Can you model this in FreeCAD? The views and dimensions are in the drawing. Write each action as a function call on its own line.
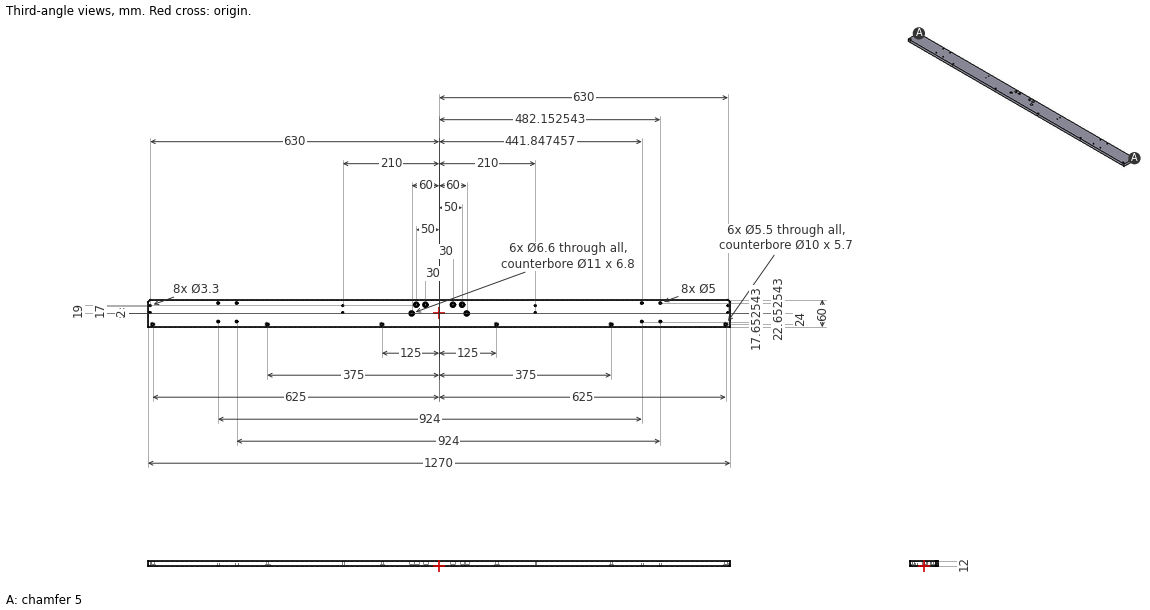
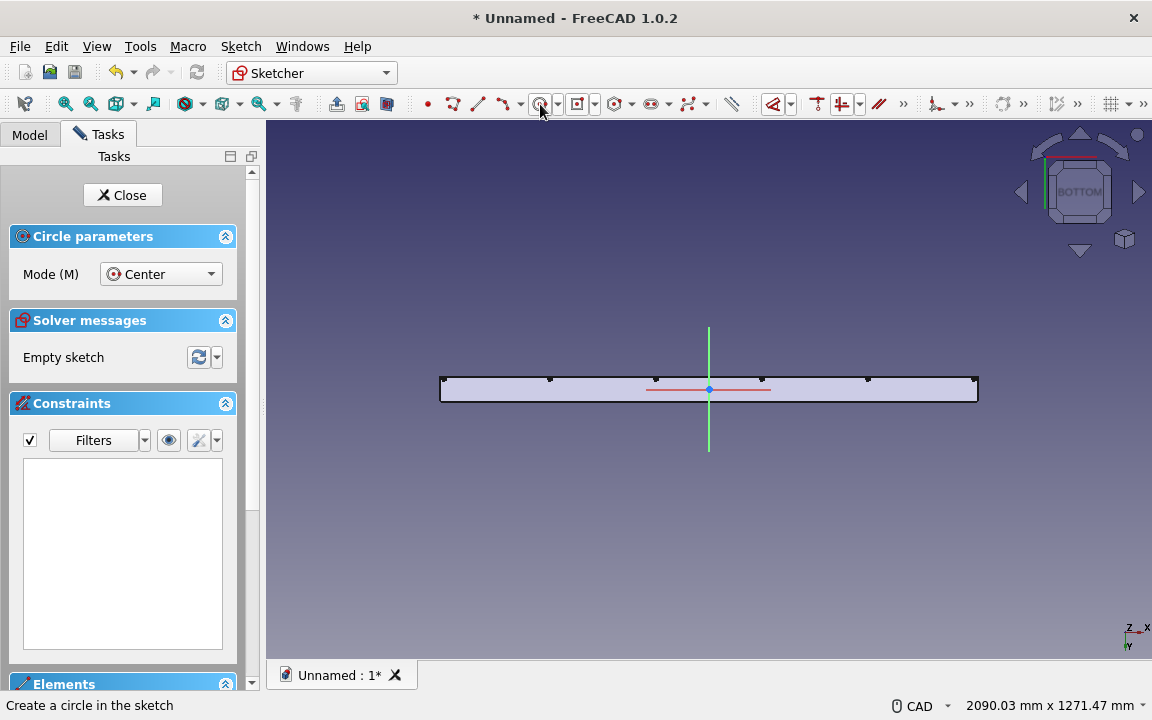
scroll(913, 399, up, 16)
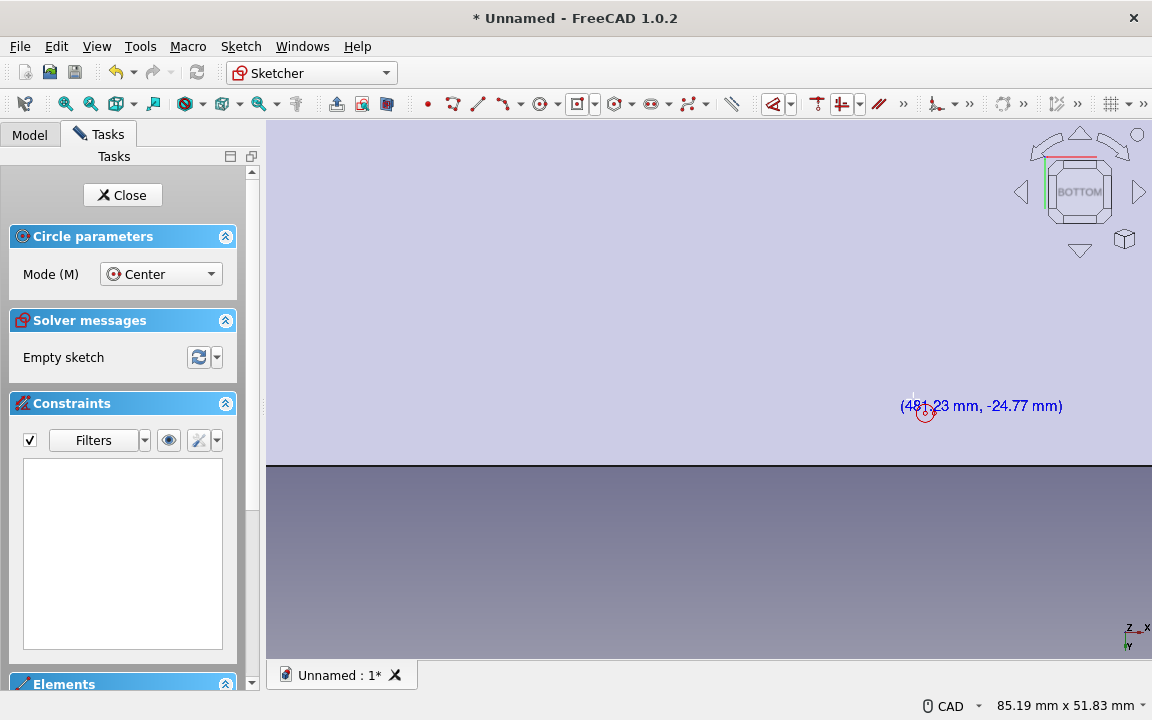
scroll(889, 400, down, 15)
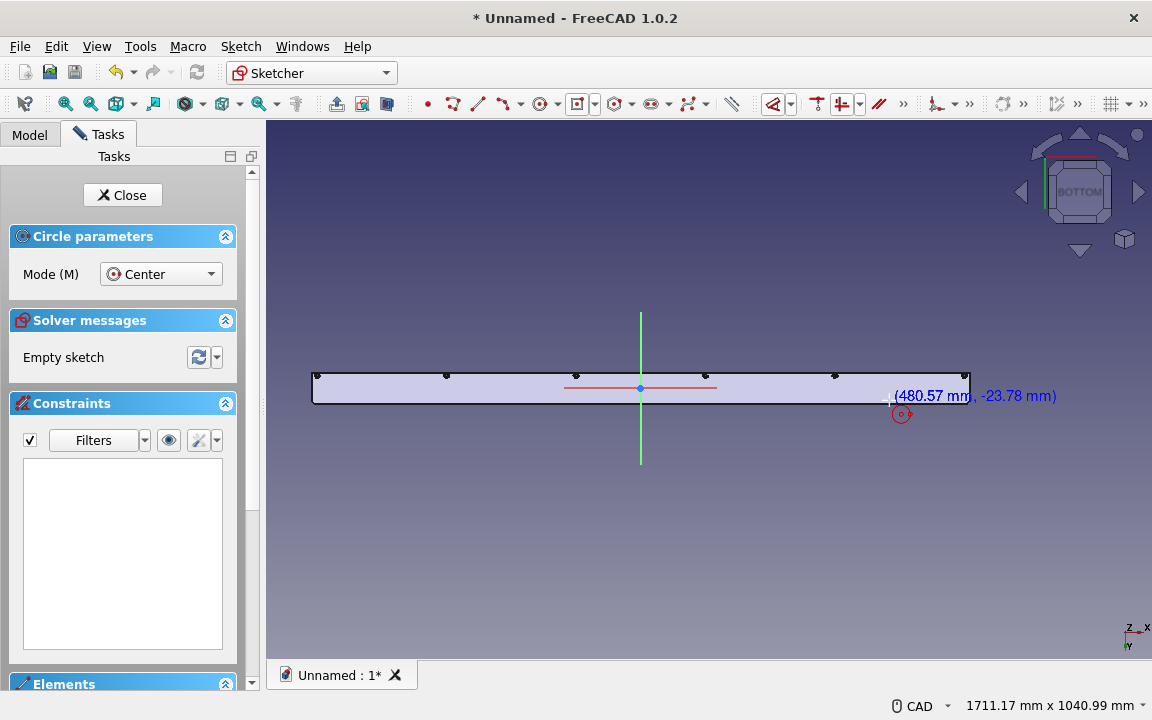
scroll(890, 400, up, 2)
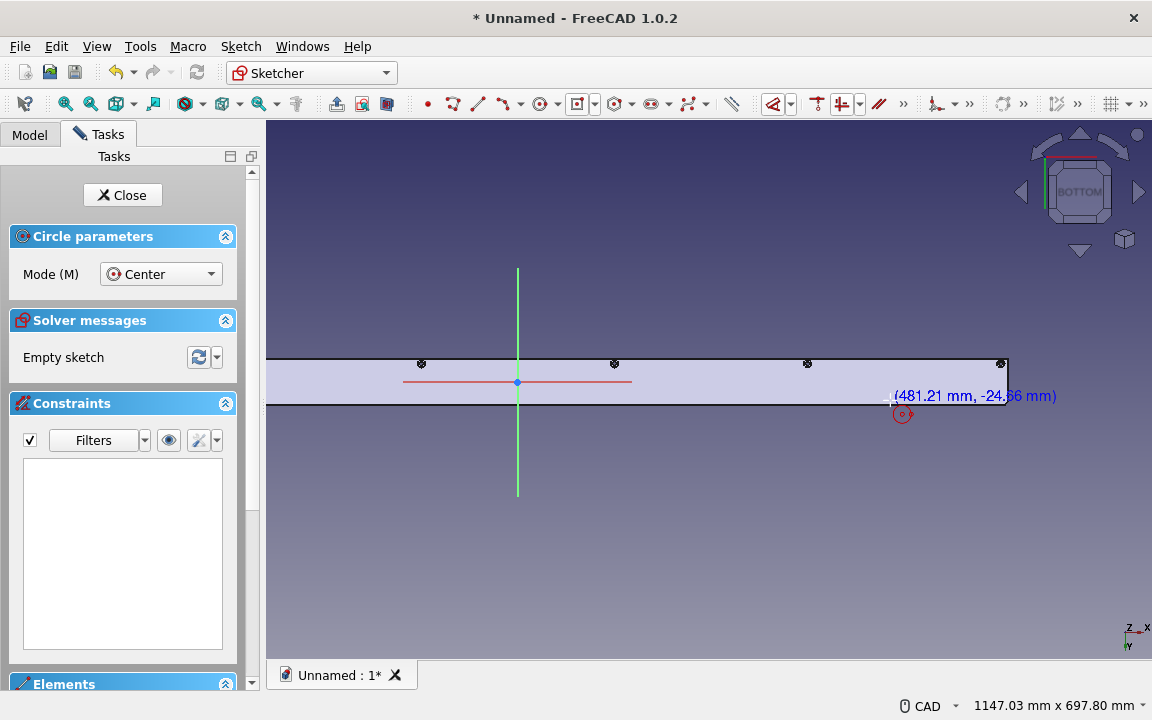
click(890, 400)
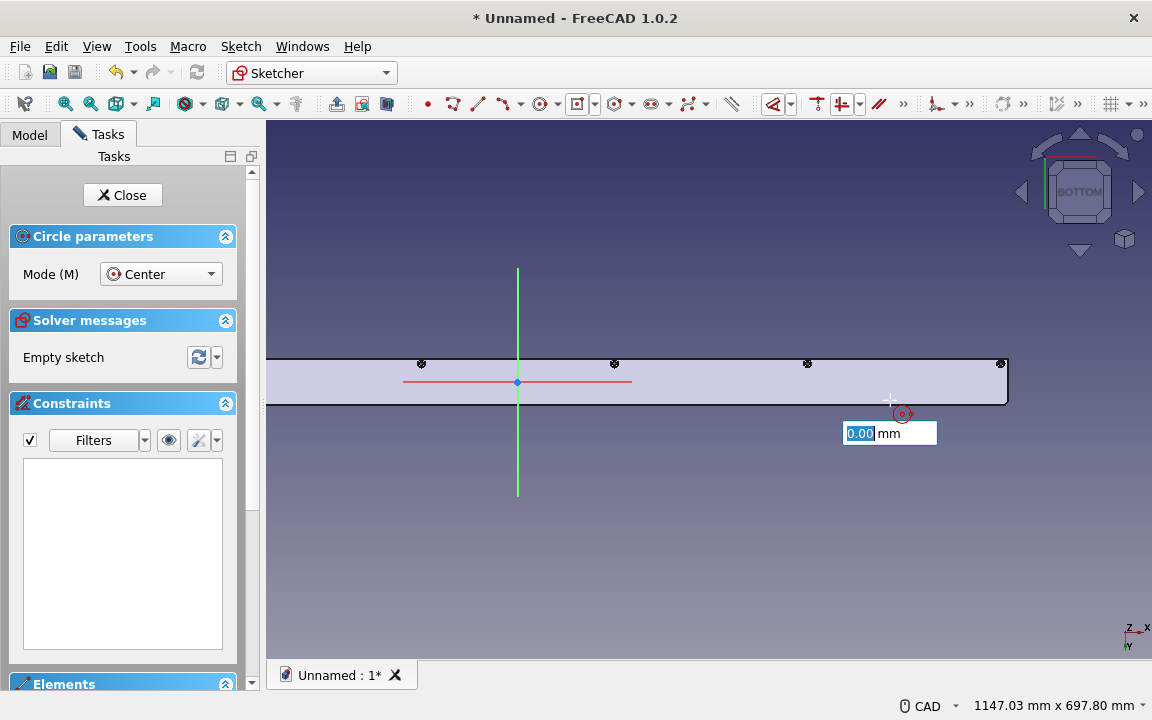
scroll(892, 398, up, 11)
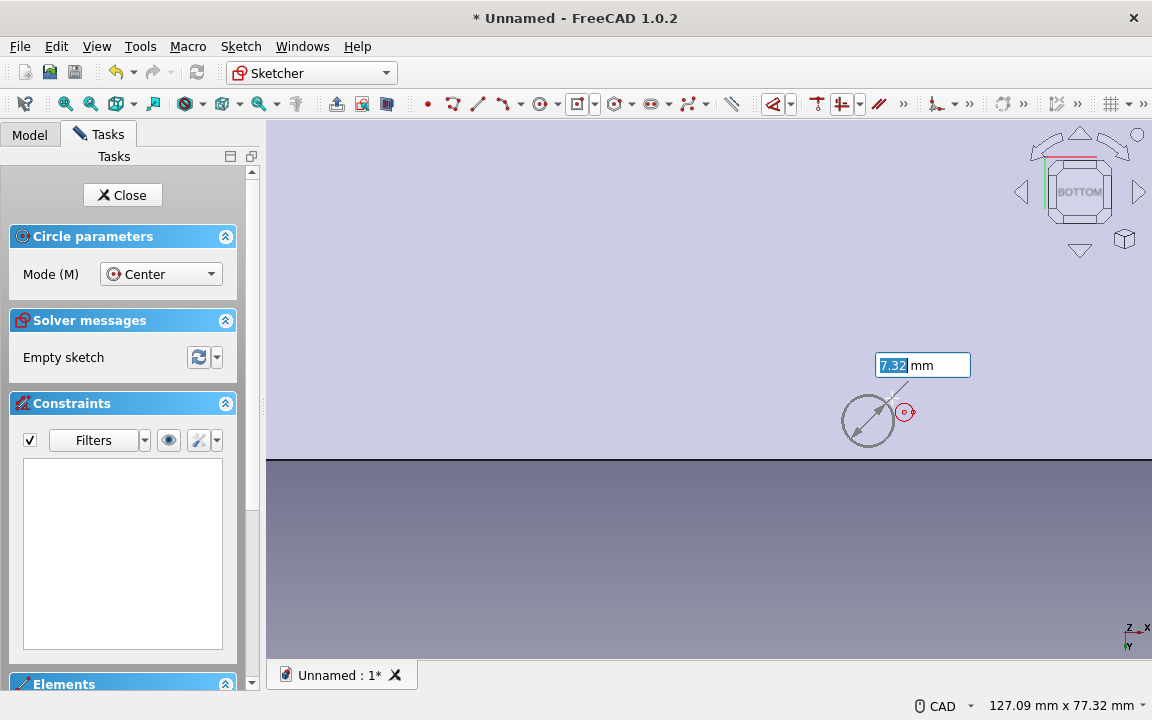
click(884, 397)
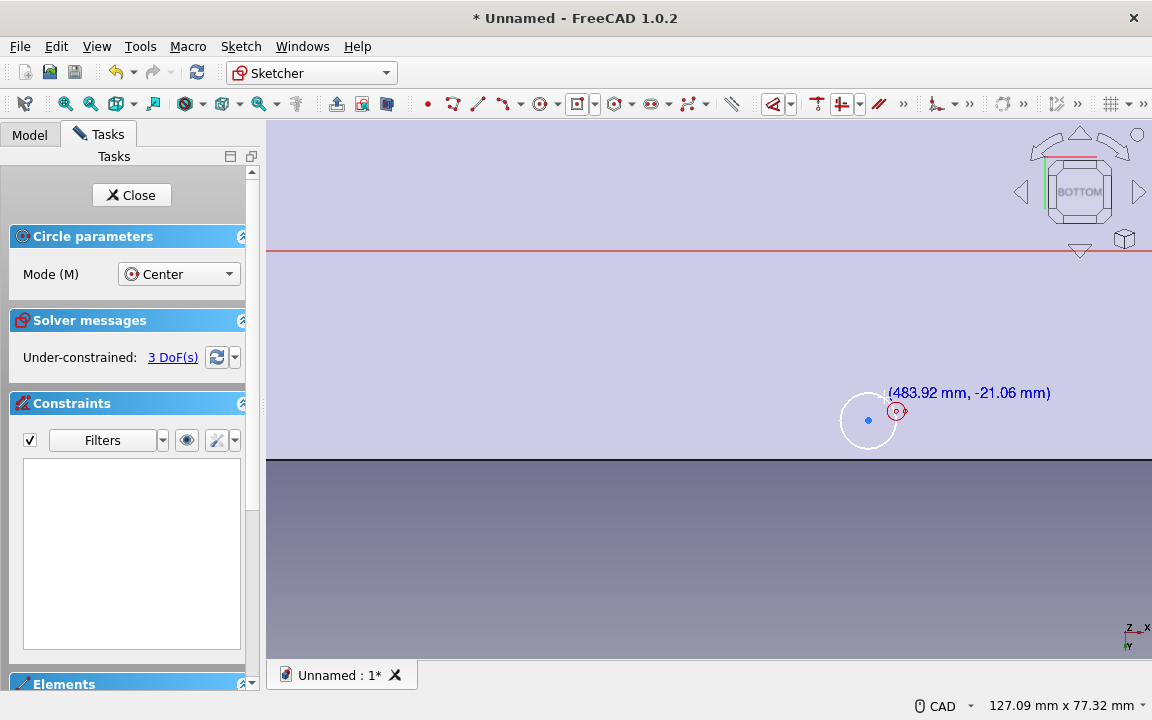
scroll(591, 409, up, 2)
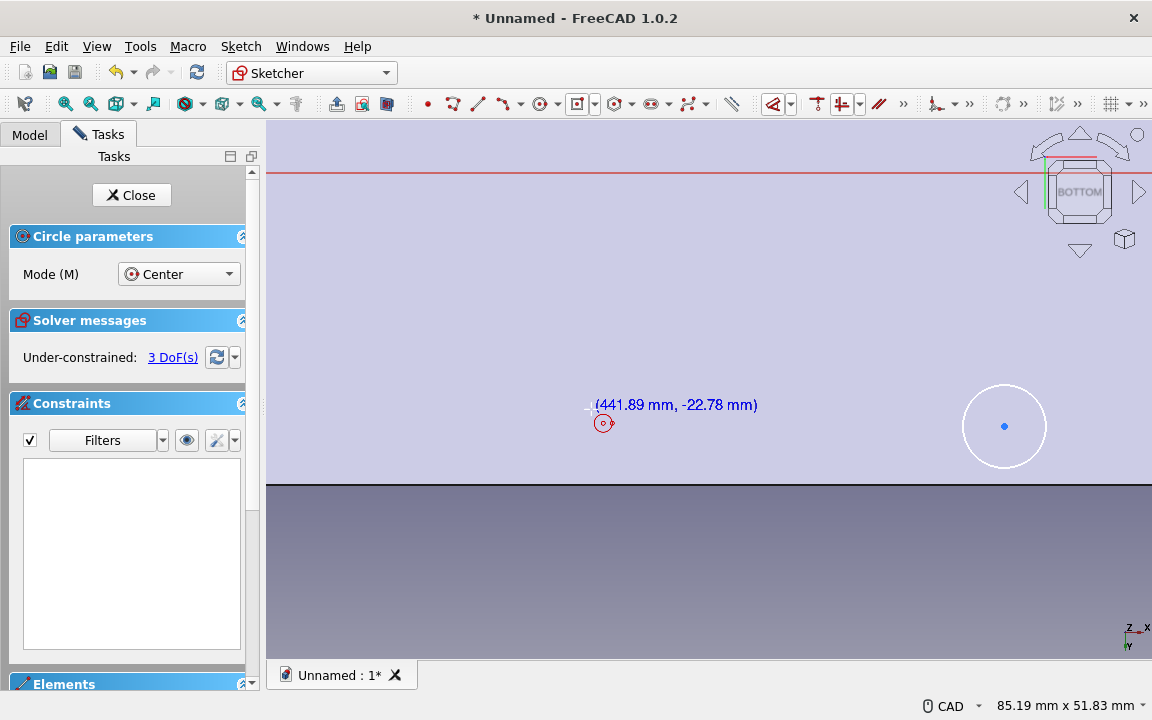
scroll(884, 399, down, 15)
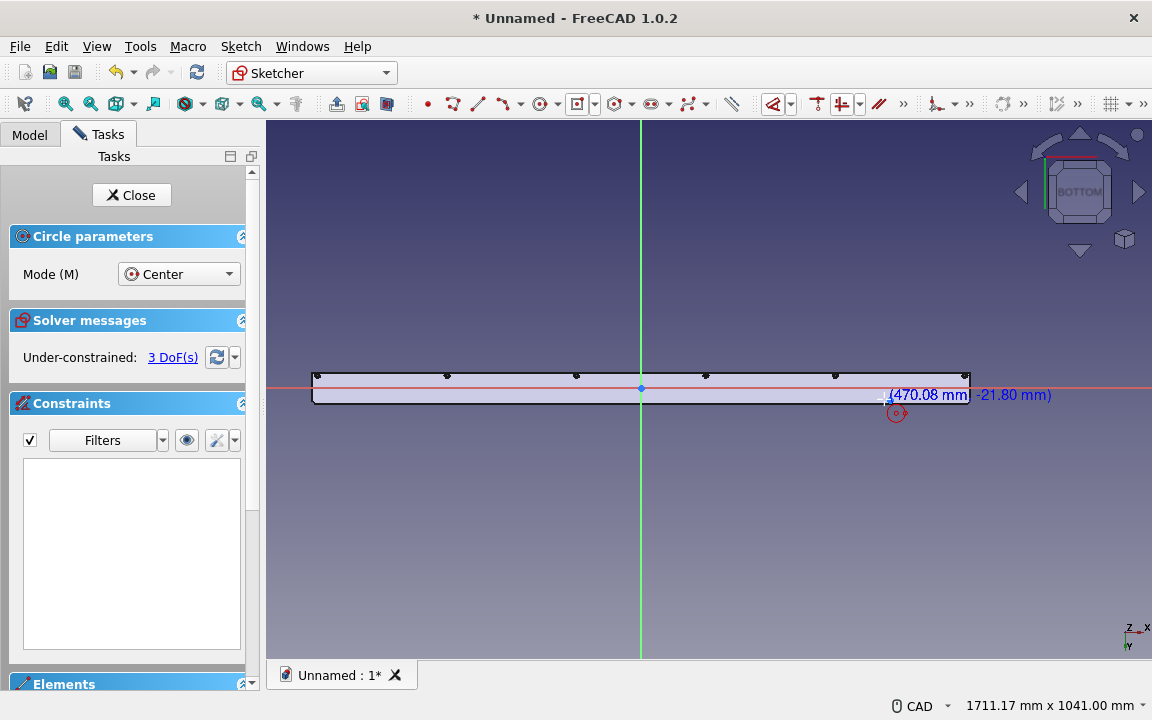
scroll(870, 400, up, 2)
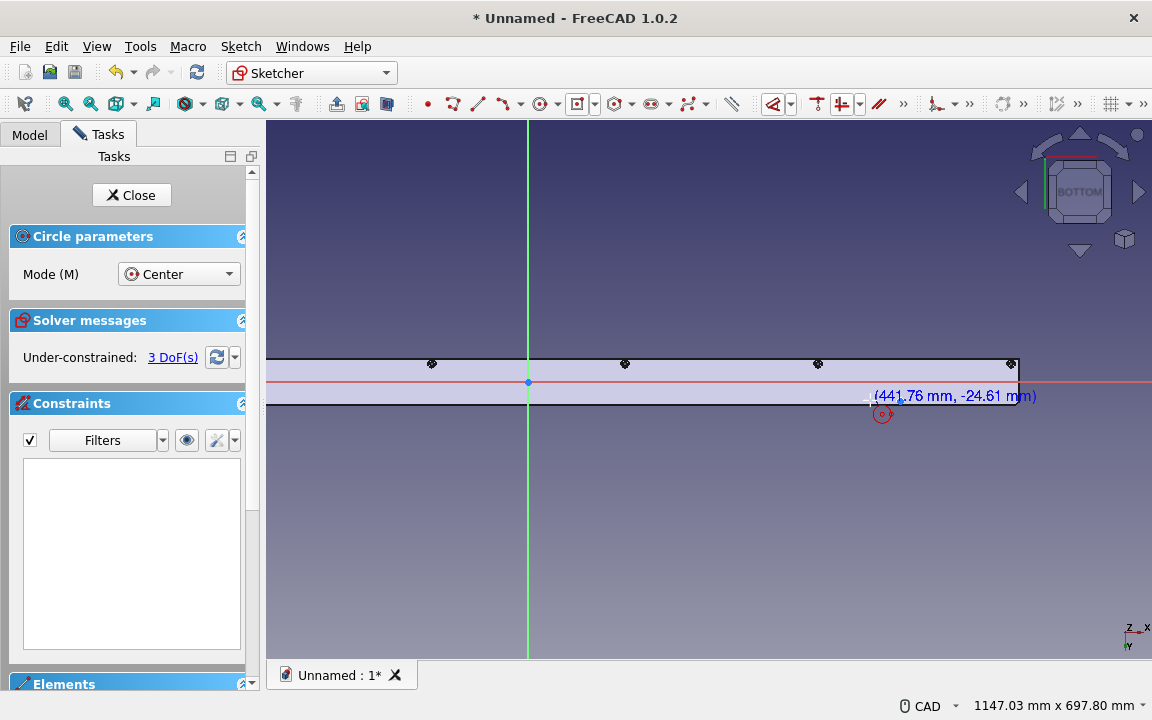
click(870, 400)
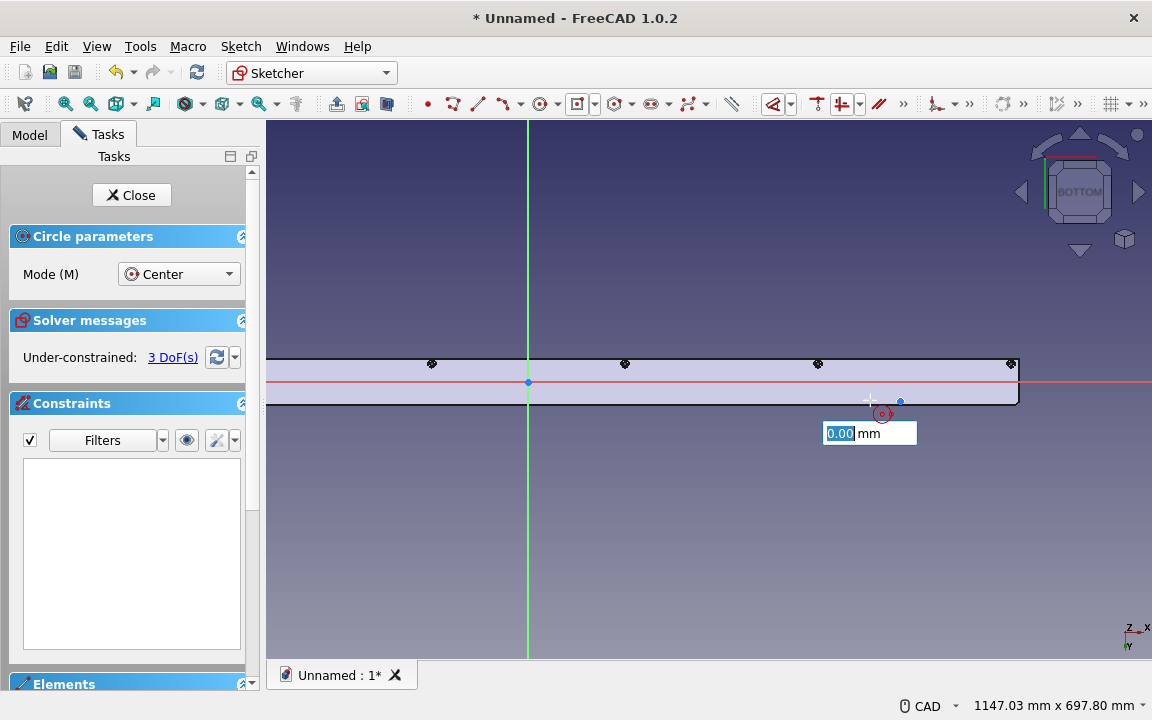
scroll(871, 398, up, 11)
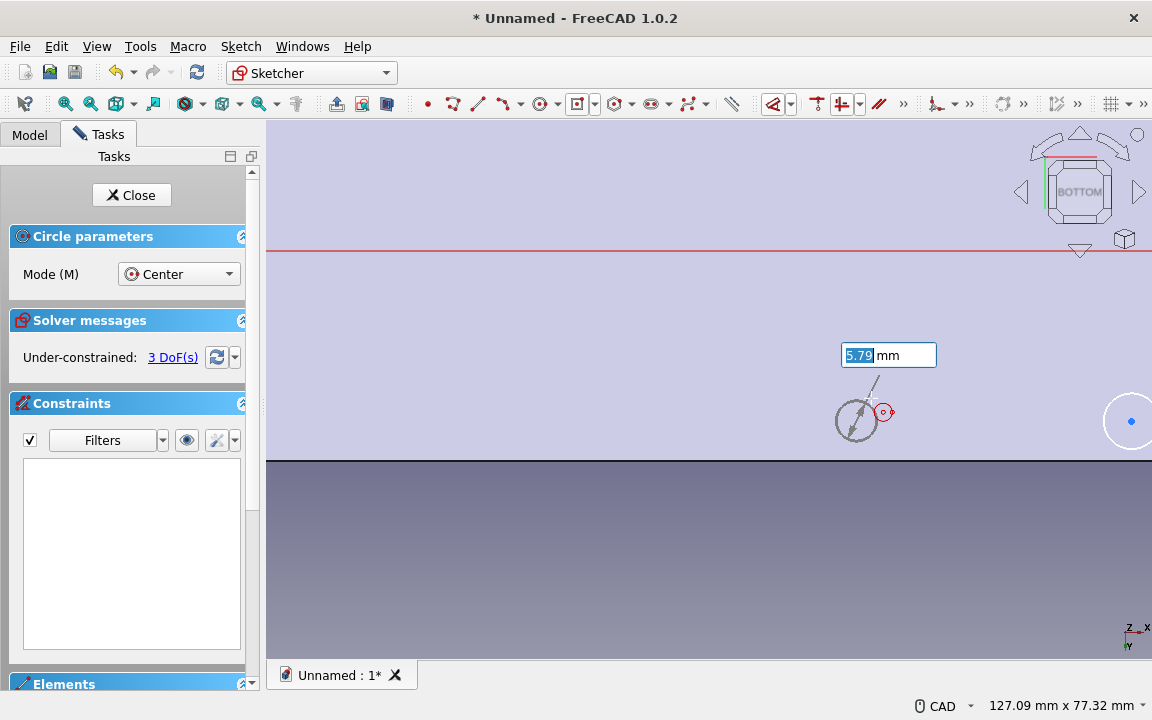
click(866, 397)